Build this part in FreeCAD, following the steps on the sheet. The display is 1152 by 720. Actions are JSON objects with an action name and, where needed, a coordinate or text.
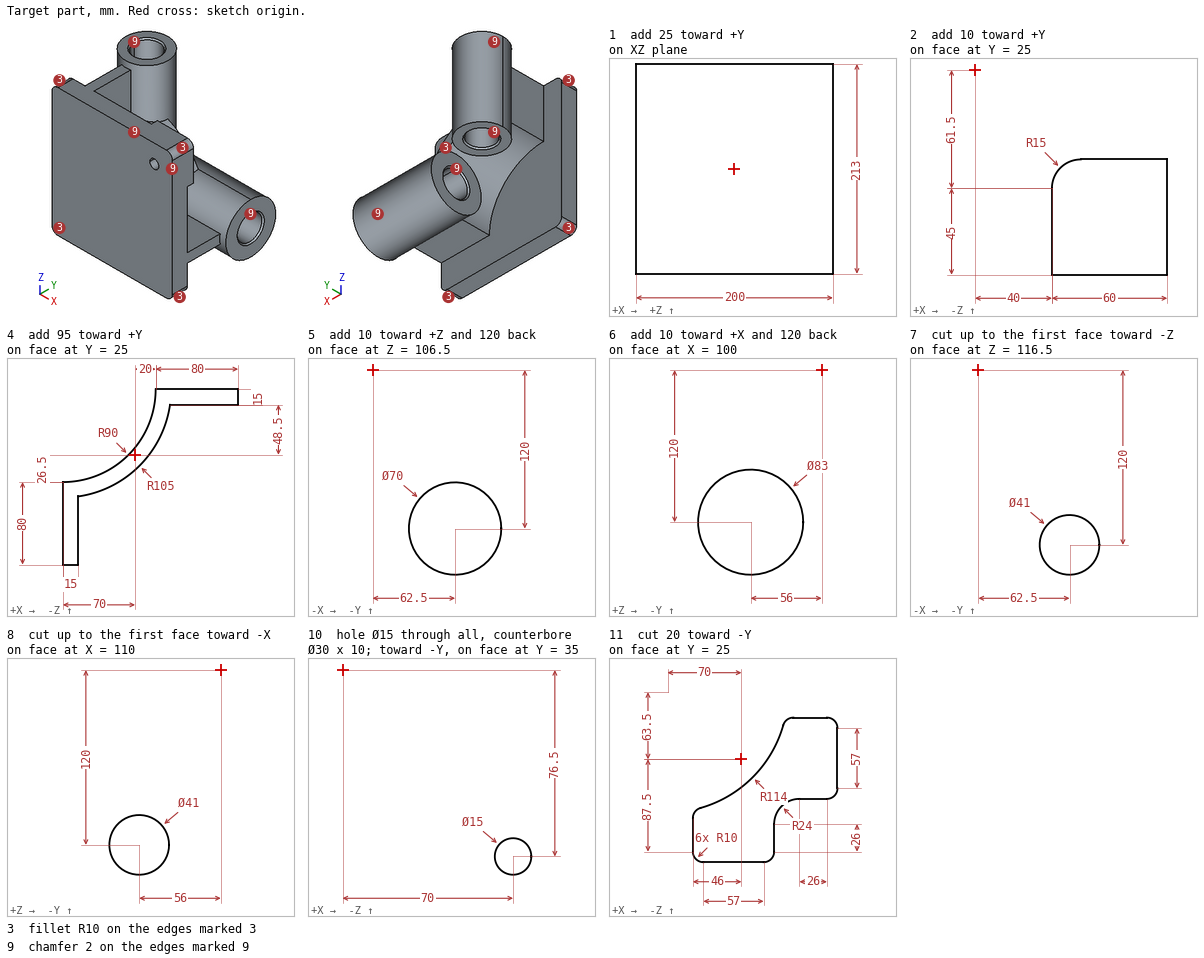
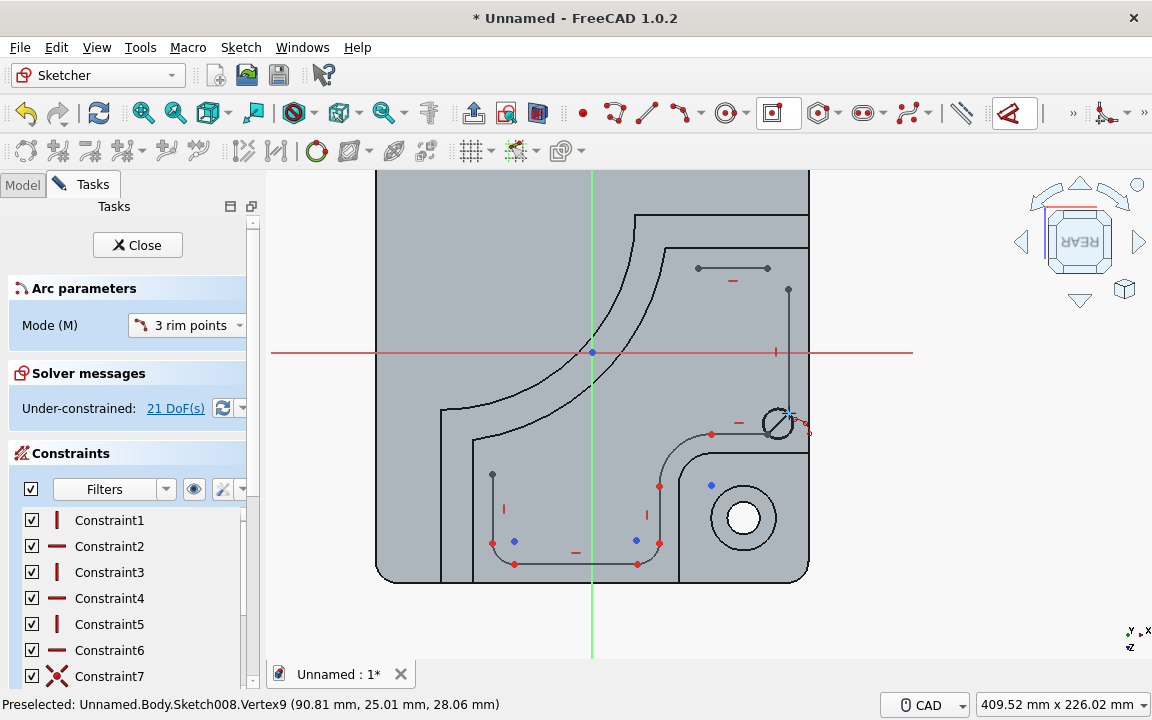
{"action": "scroll", "coordinate": [783, 427], "scroll_direction": "up", "scroll_amount": 5}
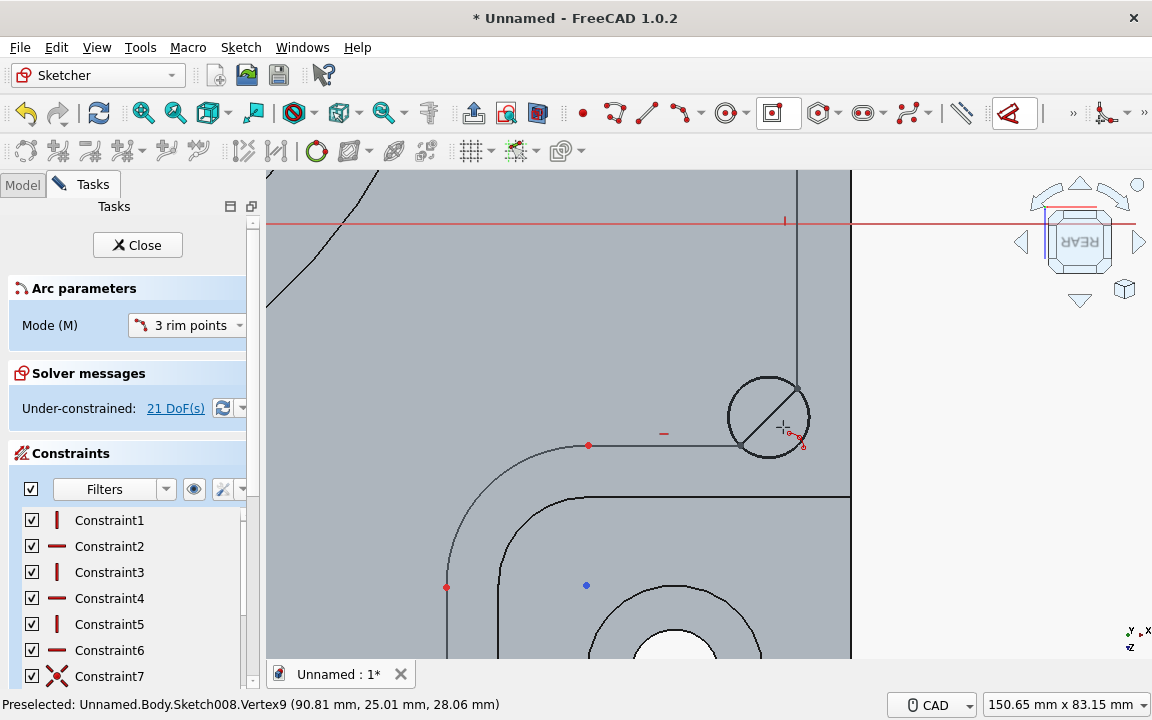
{"action": "left_click", "coordinate": [781, 427]}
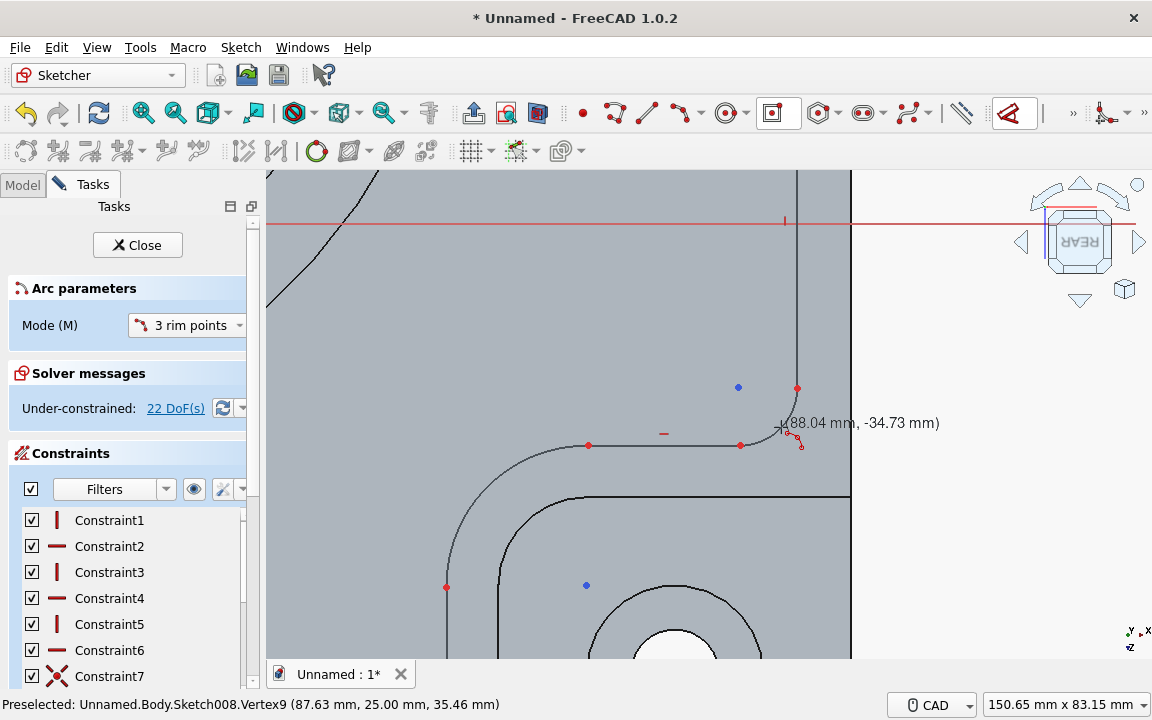
{"action": "scroll", "coordinate": [783, 426], "scroll_direction": "down", "scroll_amount": 5}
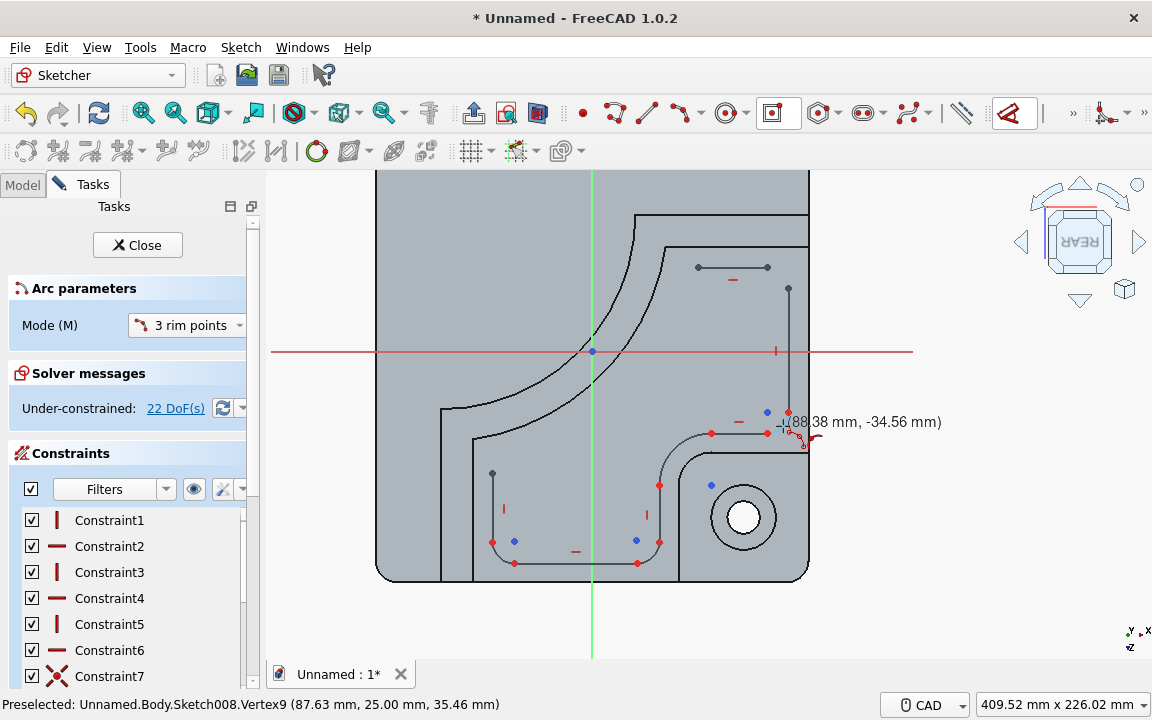
{"action": "left_click", "coordinate": [789, 289]}
{"action": "left_click", "coordinate": [768, 268]}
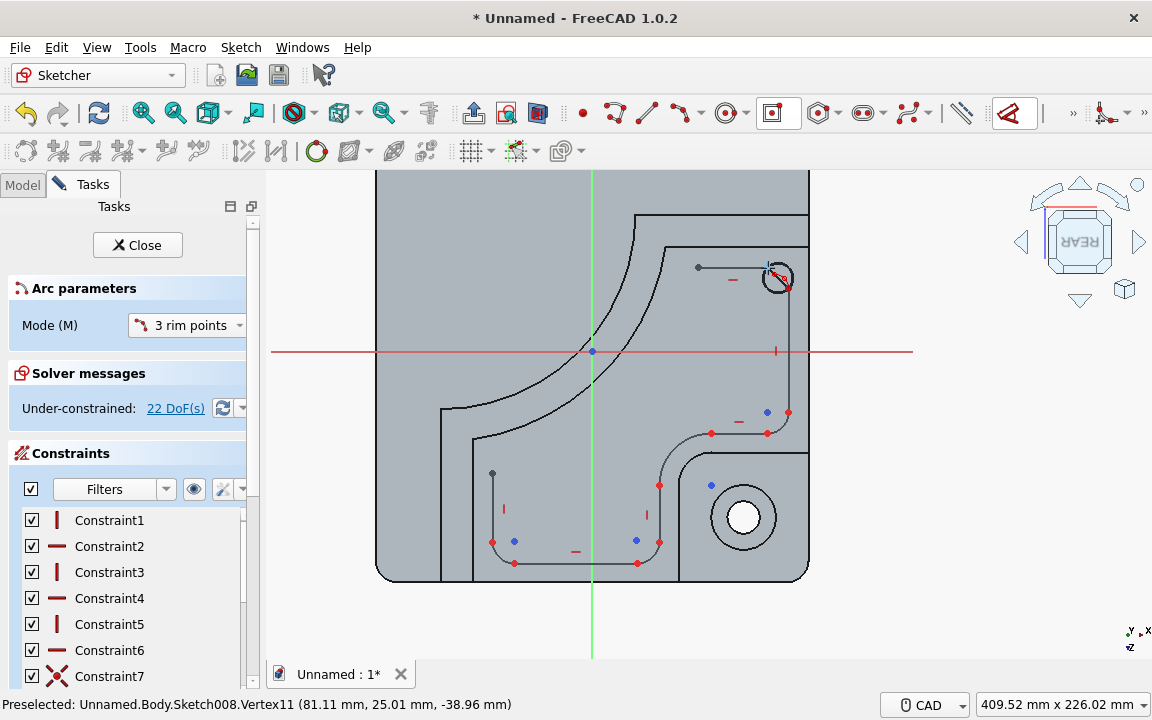
{"action": "scroll", "coordinate": [783, 273], "scroll_direction": "up", "scroll_amount": 5}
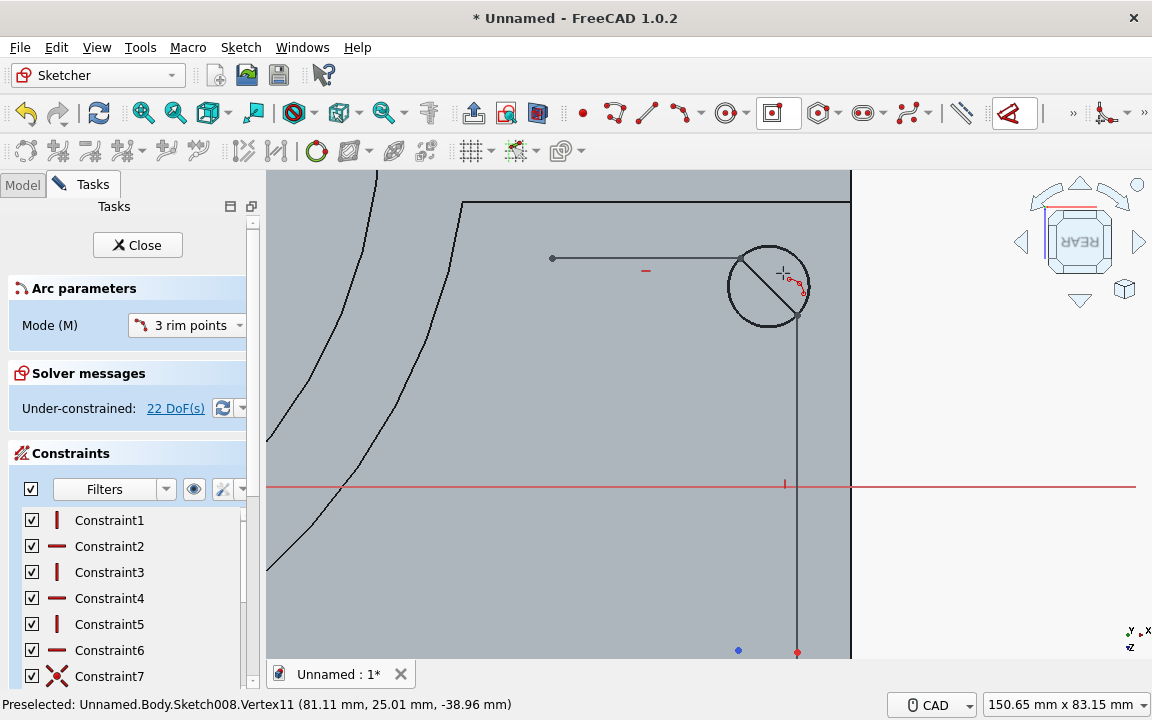
{"action": "left_click", "coordinate": [781, 272]}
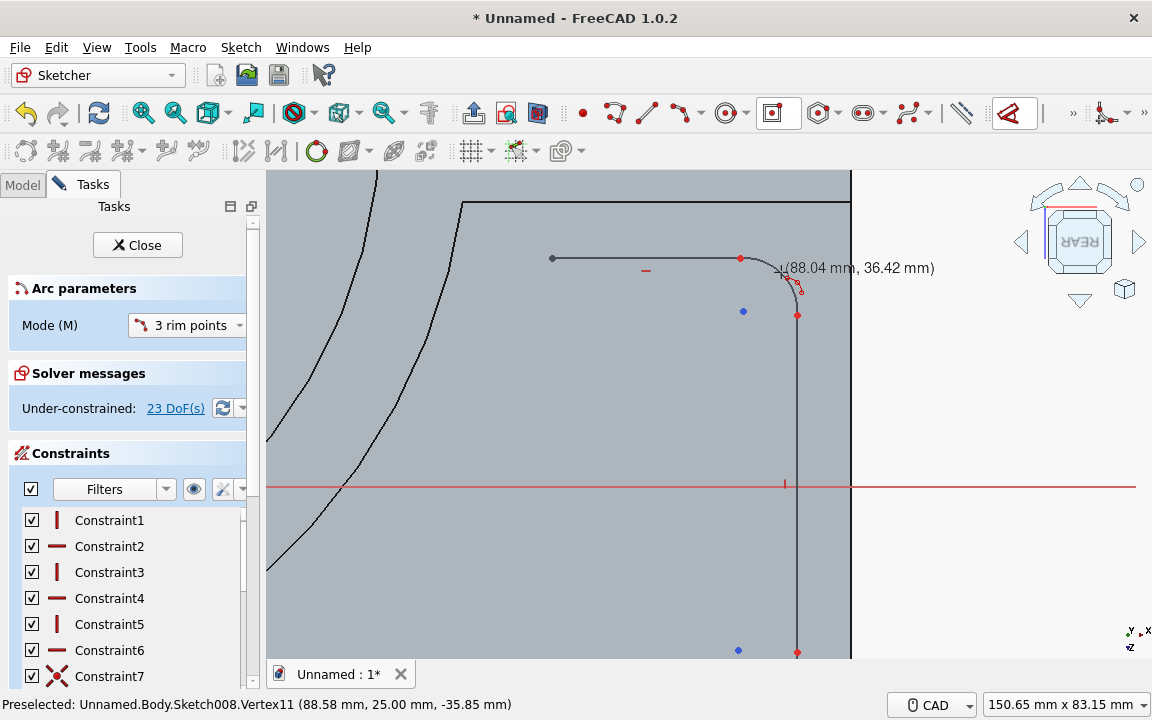
{"action": "left_click", "coordinate": [553, 258]}
{"action": "left_click", "coordinate": [496, 298]}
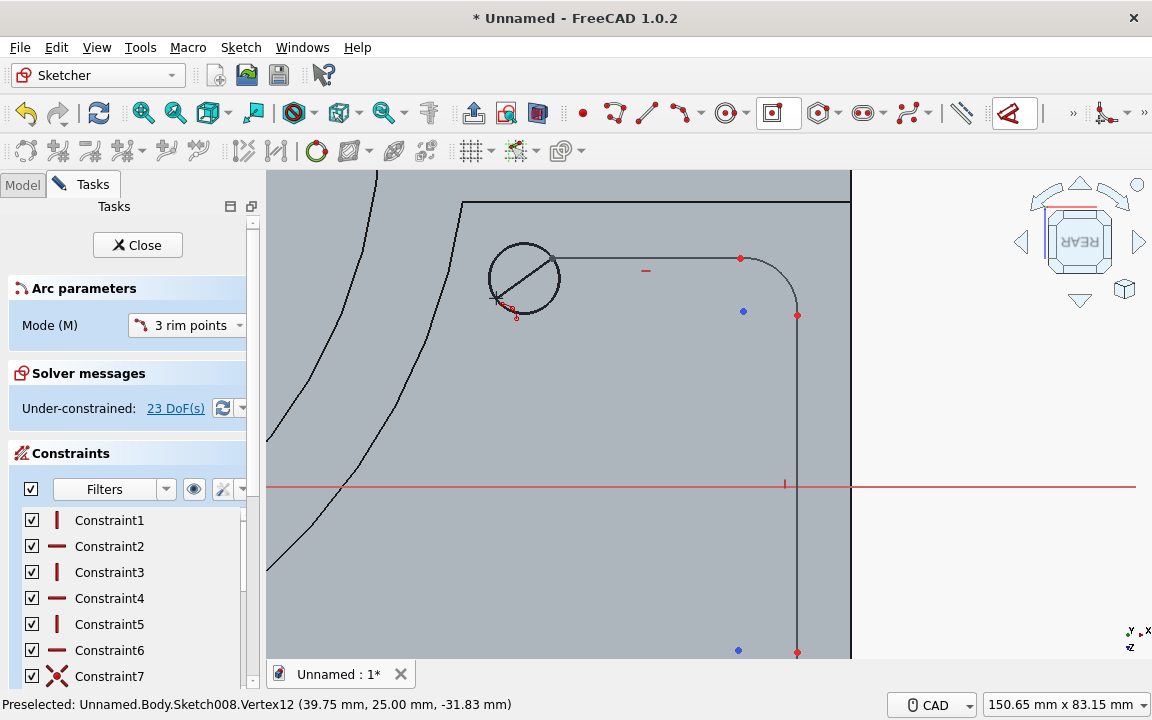
{"action": "scroll", "coordinate": [517, 267], "scroll_direction": "up", "scroll_amount": 2}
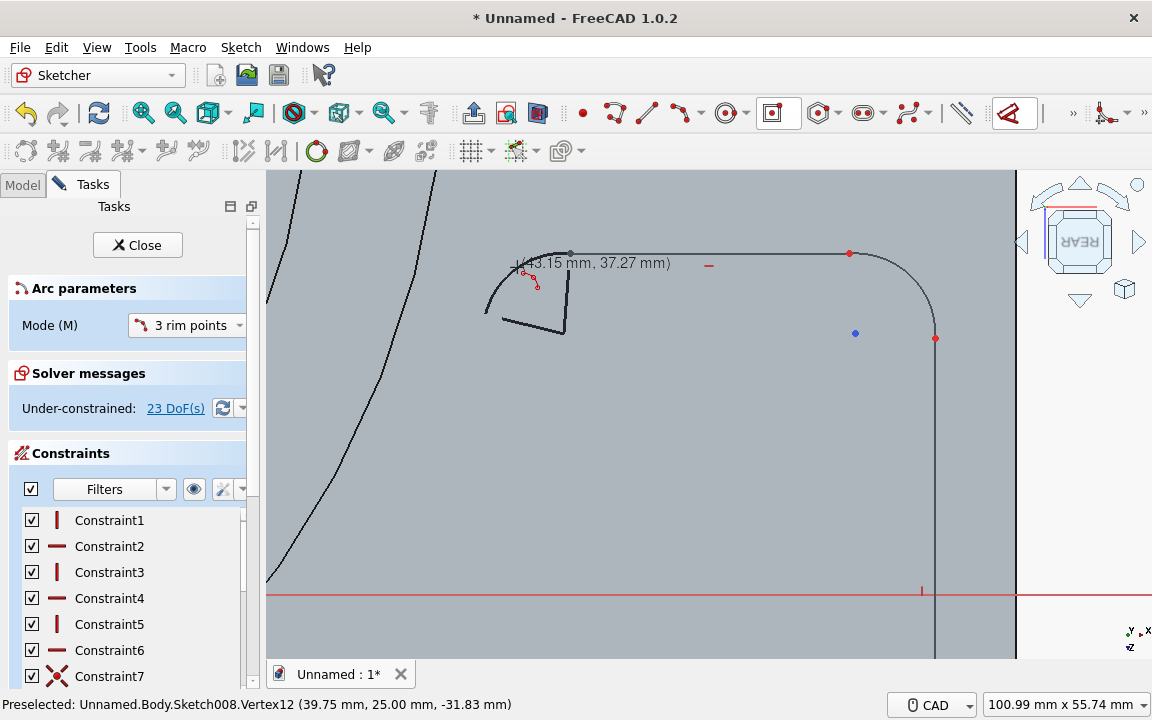
{"action": "left_click", "coordinate": [518, 267]}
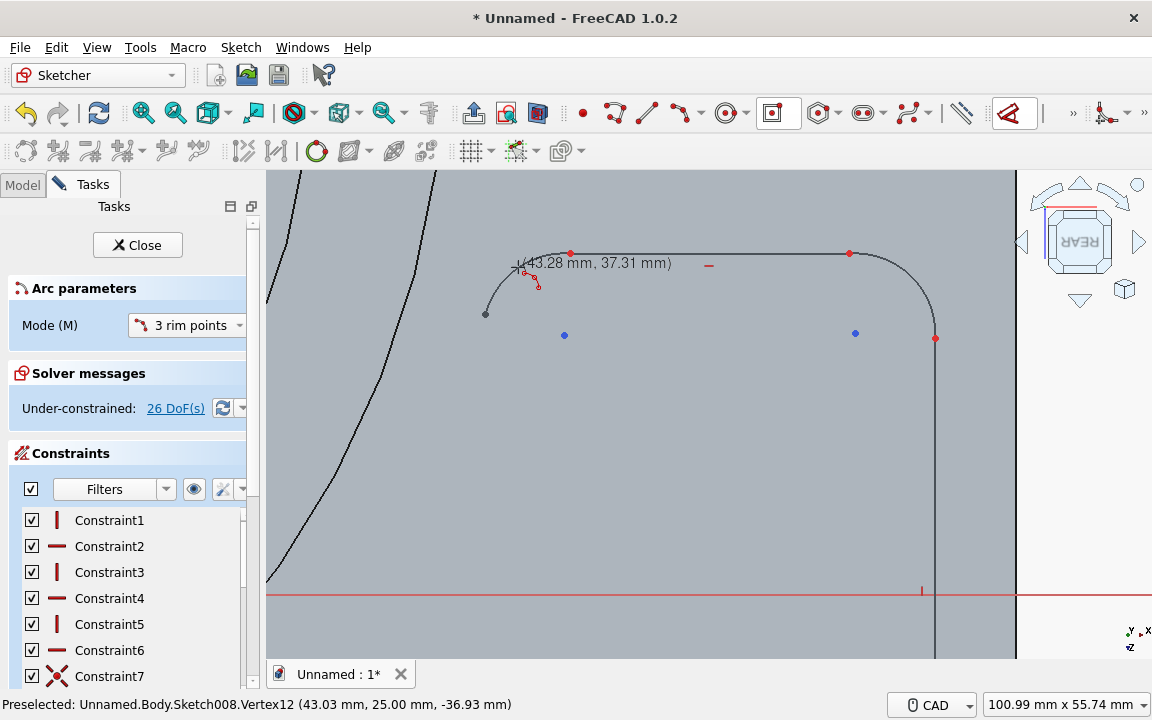
{"action": "scroll", "coordinate": [740, 272], "scroll_direction": "down", "scroll_amount": 7}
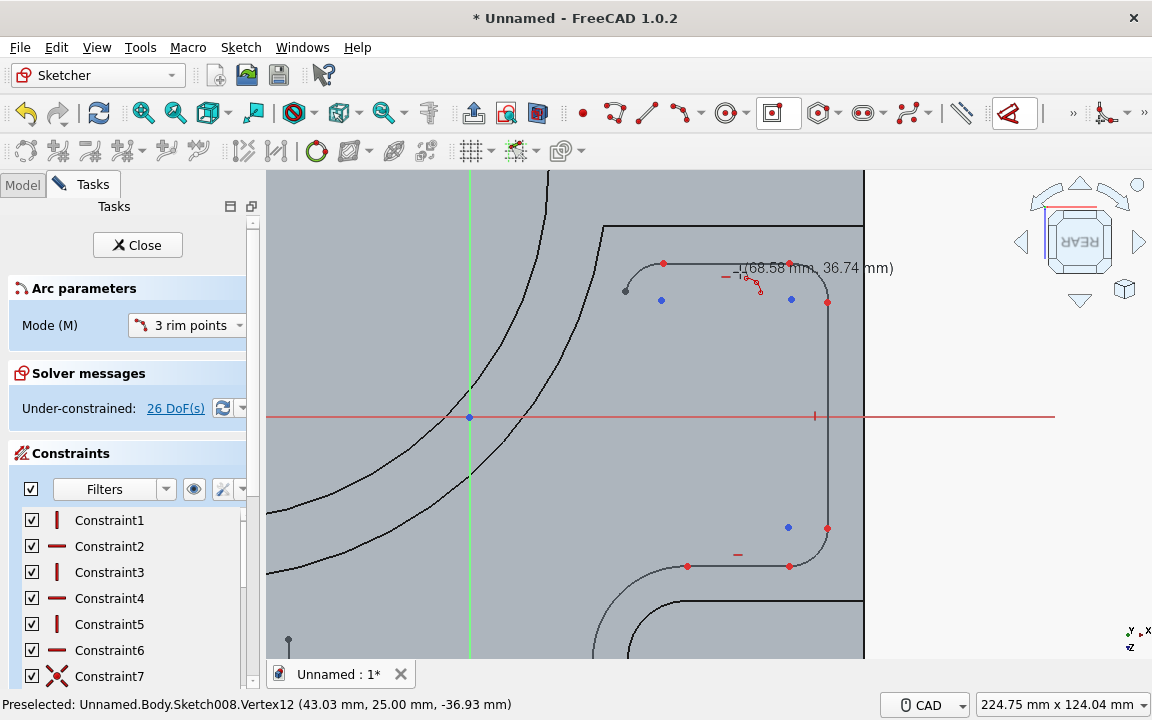
{"action": "left_click", "coordinate": [678, 283]}
{"action": "left_click", "coordinate": [508, 452]}
{"action": "left_click", "coordinate": [615, 389]}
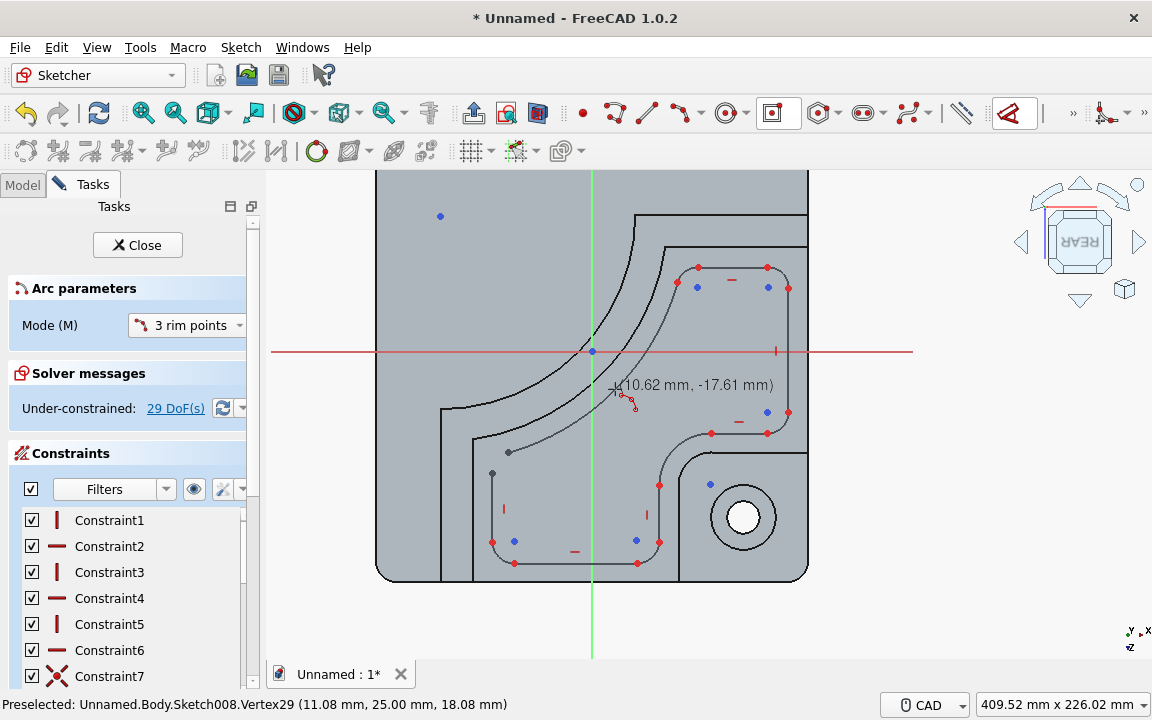
{"action": "left_click", "coordinate": [508, 453]}
{"action": "left_click", "coordinate": [492, 474]}